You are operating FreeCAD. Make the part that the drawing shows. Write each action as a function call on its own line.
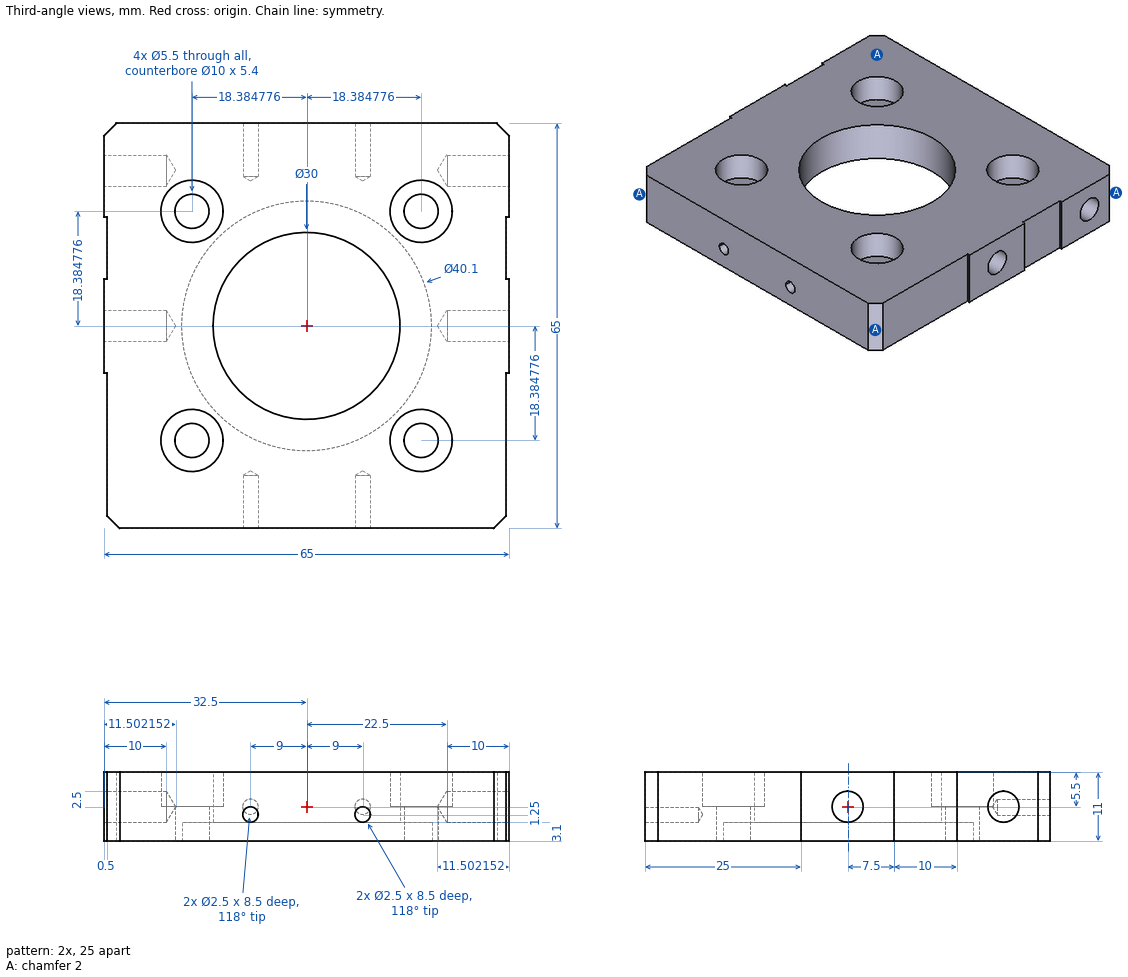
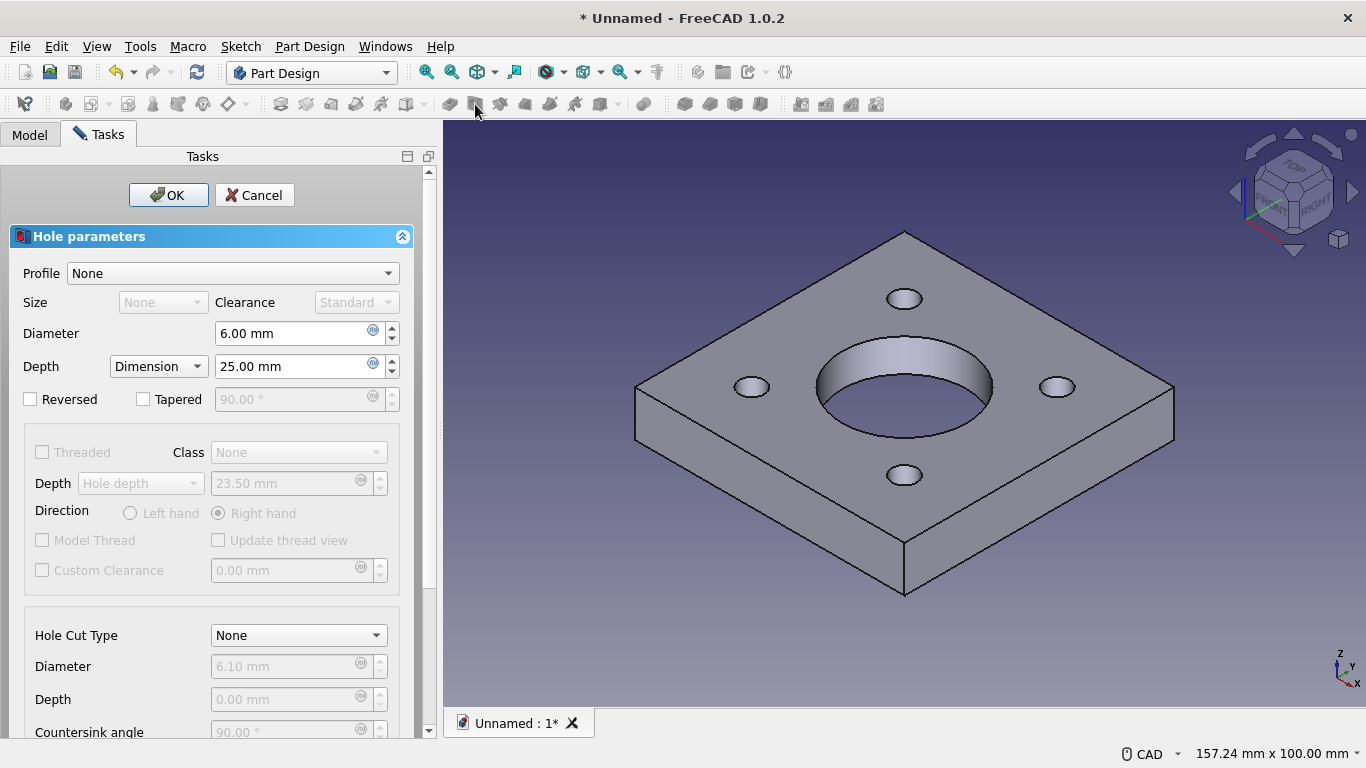
triple_click(300, 334)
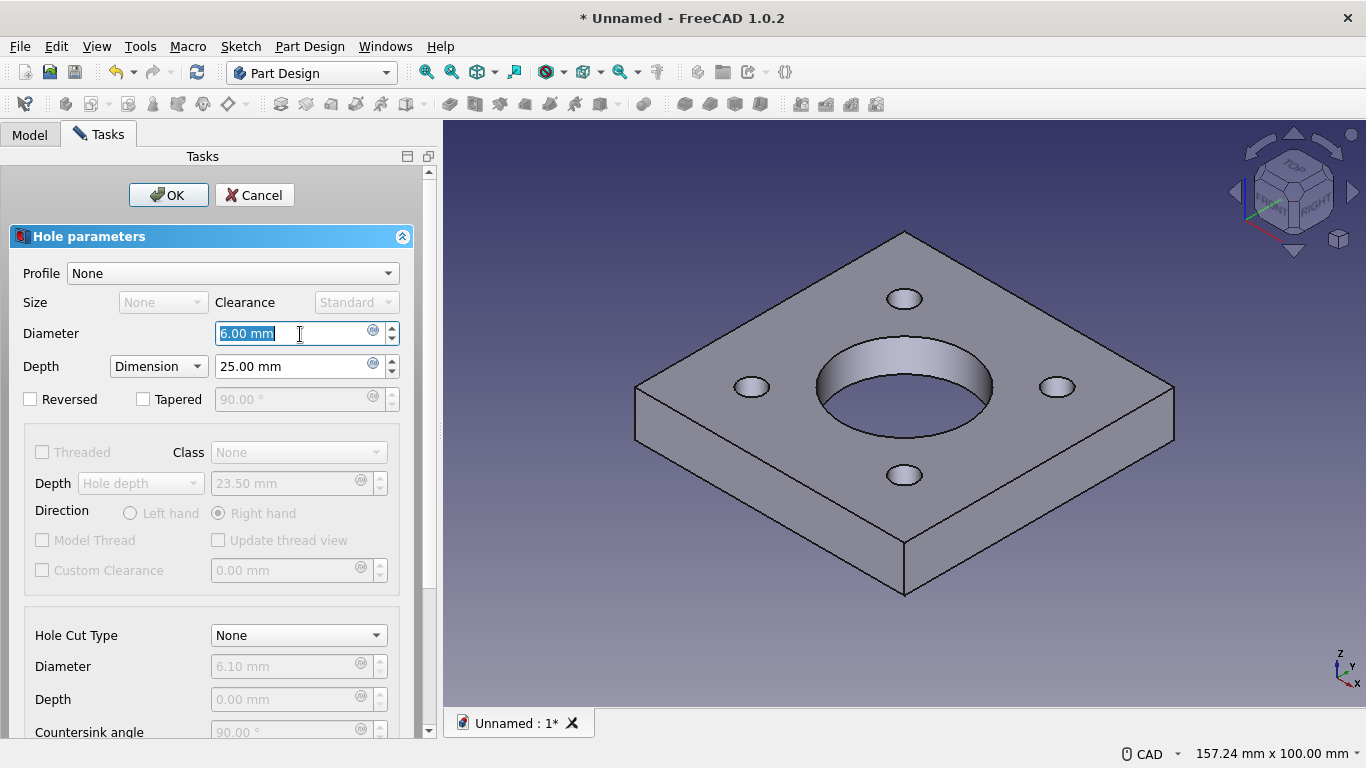
text(5.5)
key(Tab)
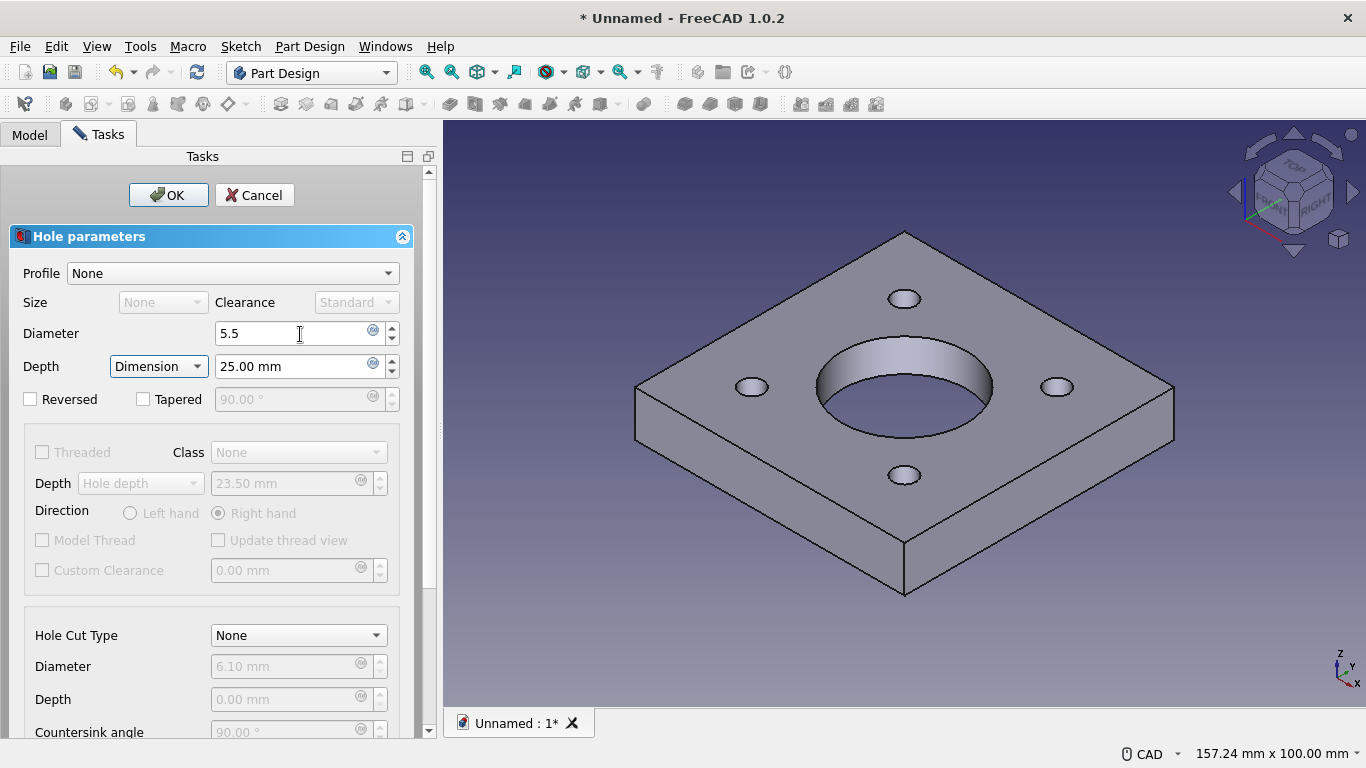
click(160, 366)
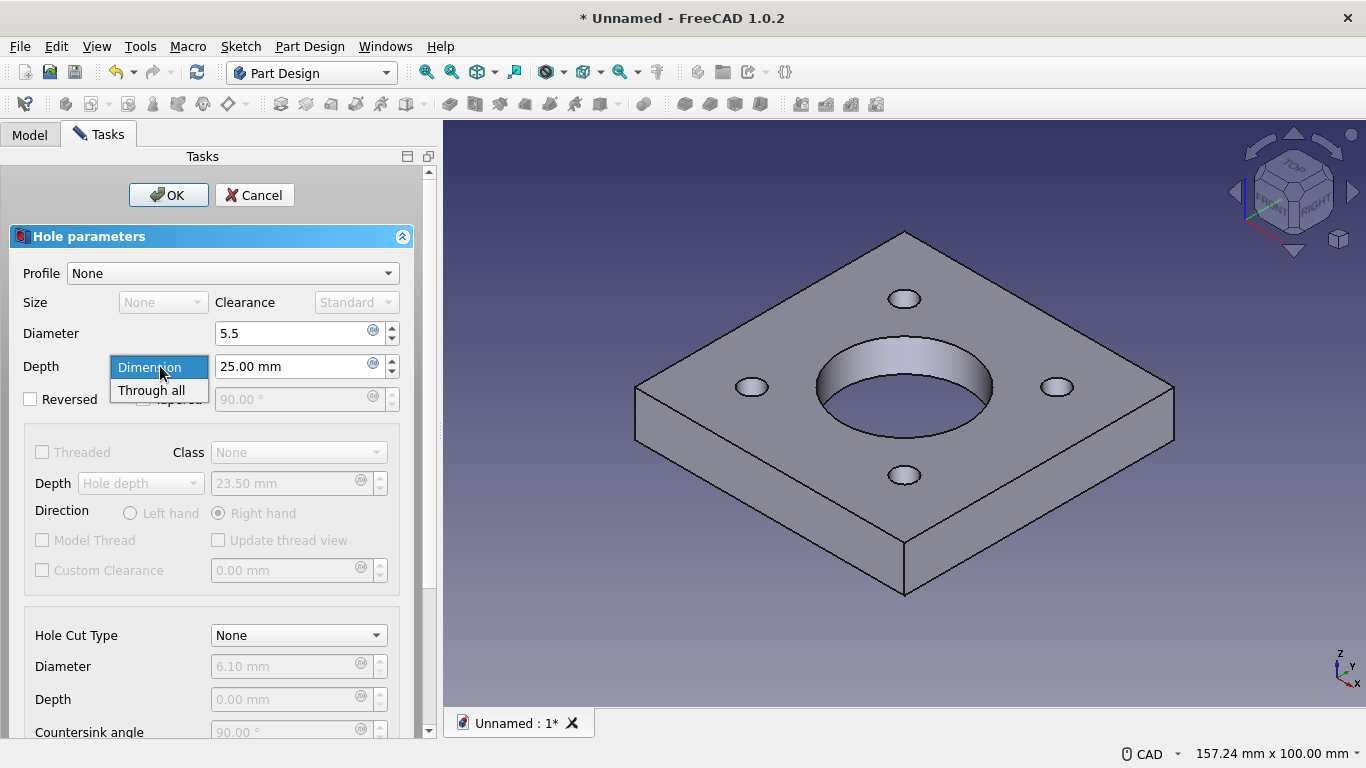
click(158, 390)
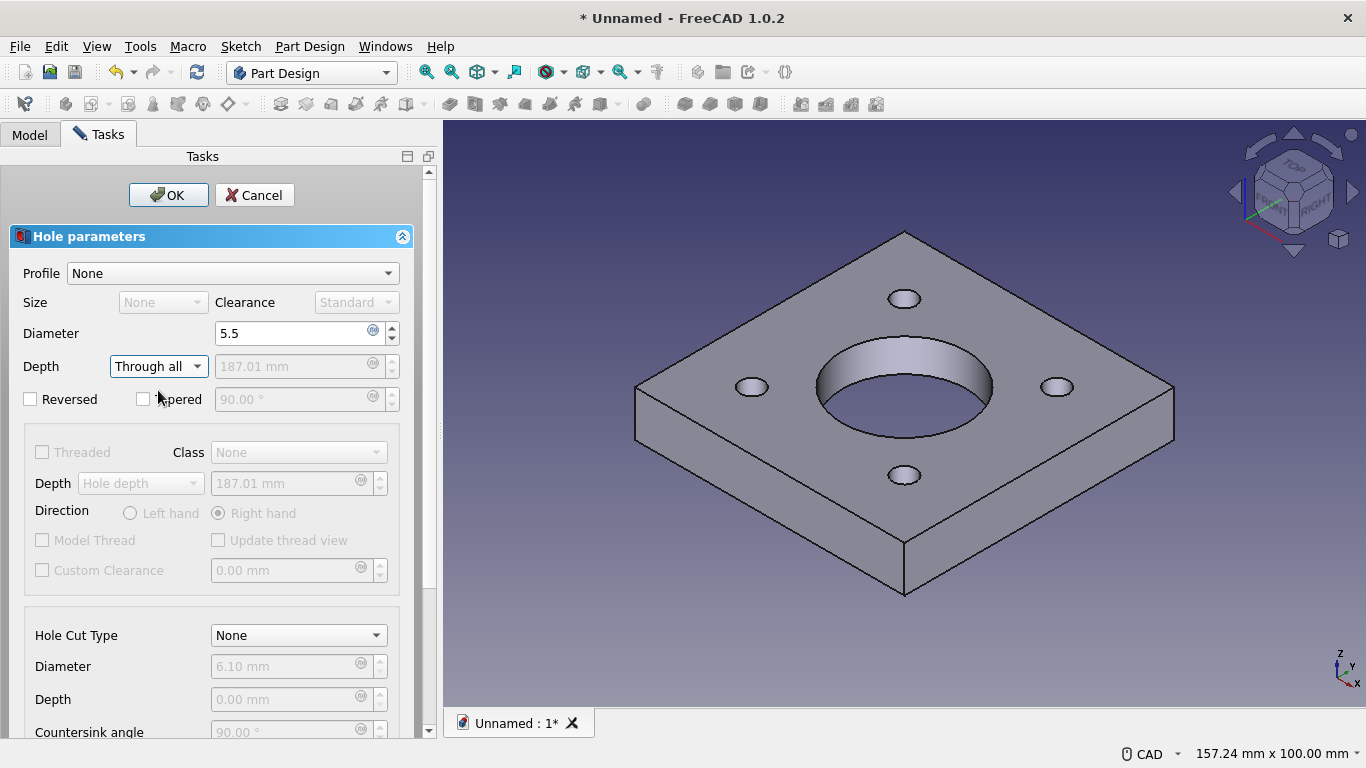
click(300, 636)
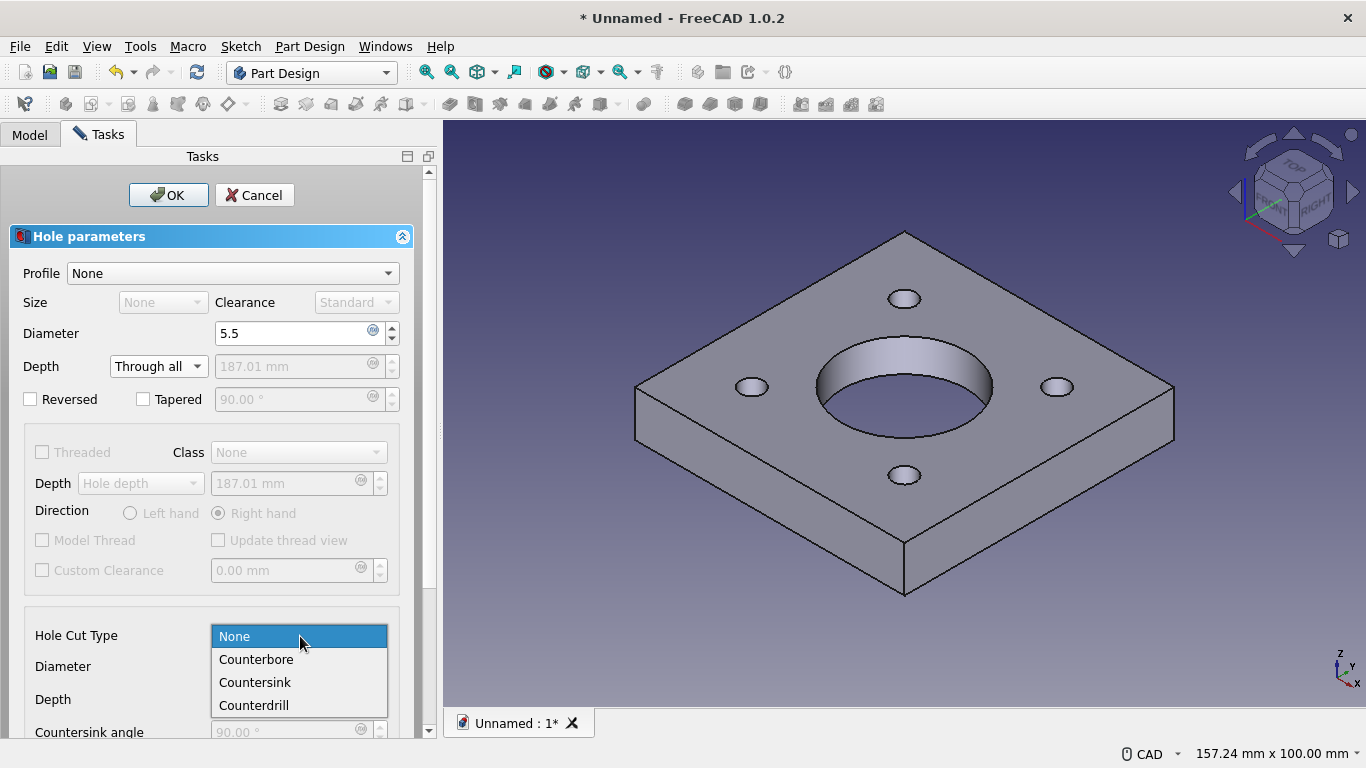
click(298, 660)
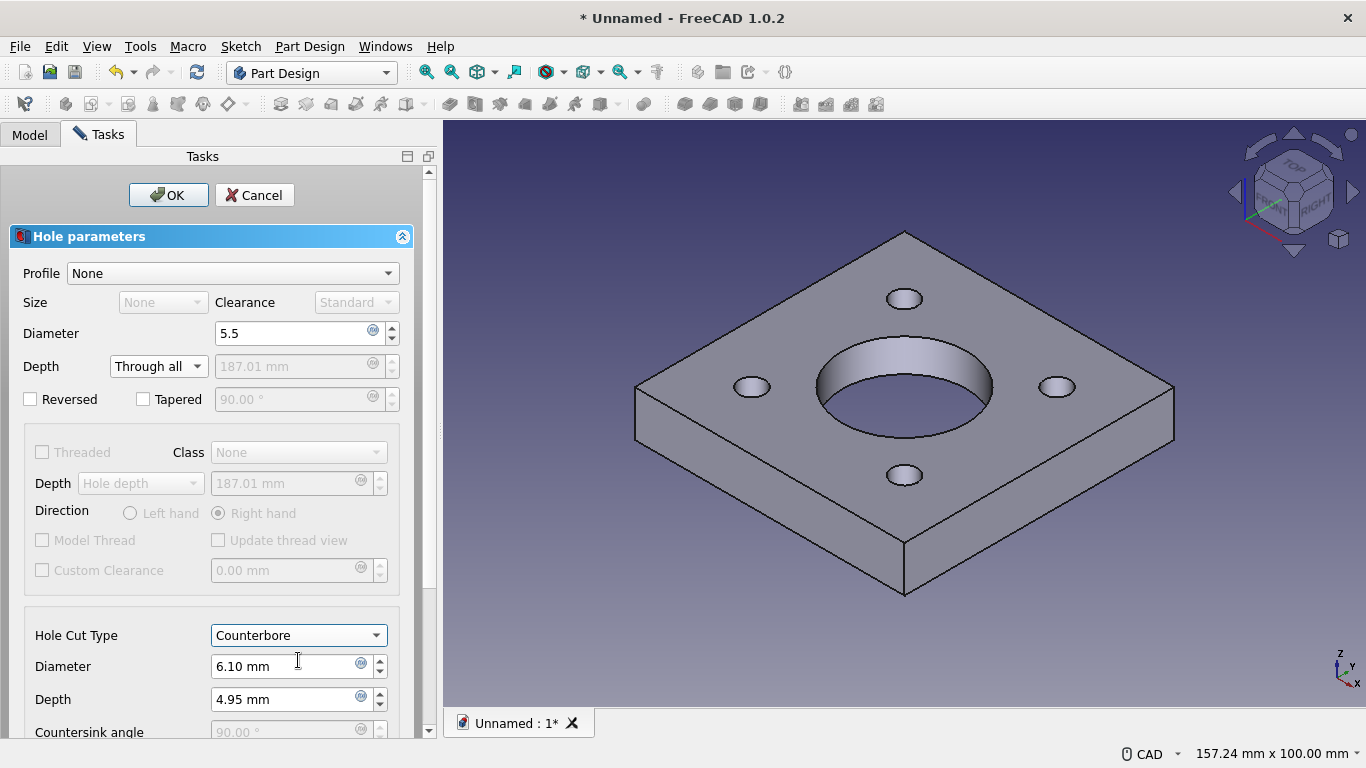
triple_click(292, 666)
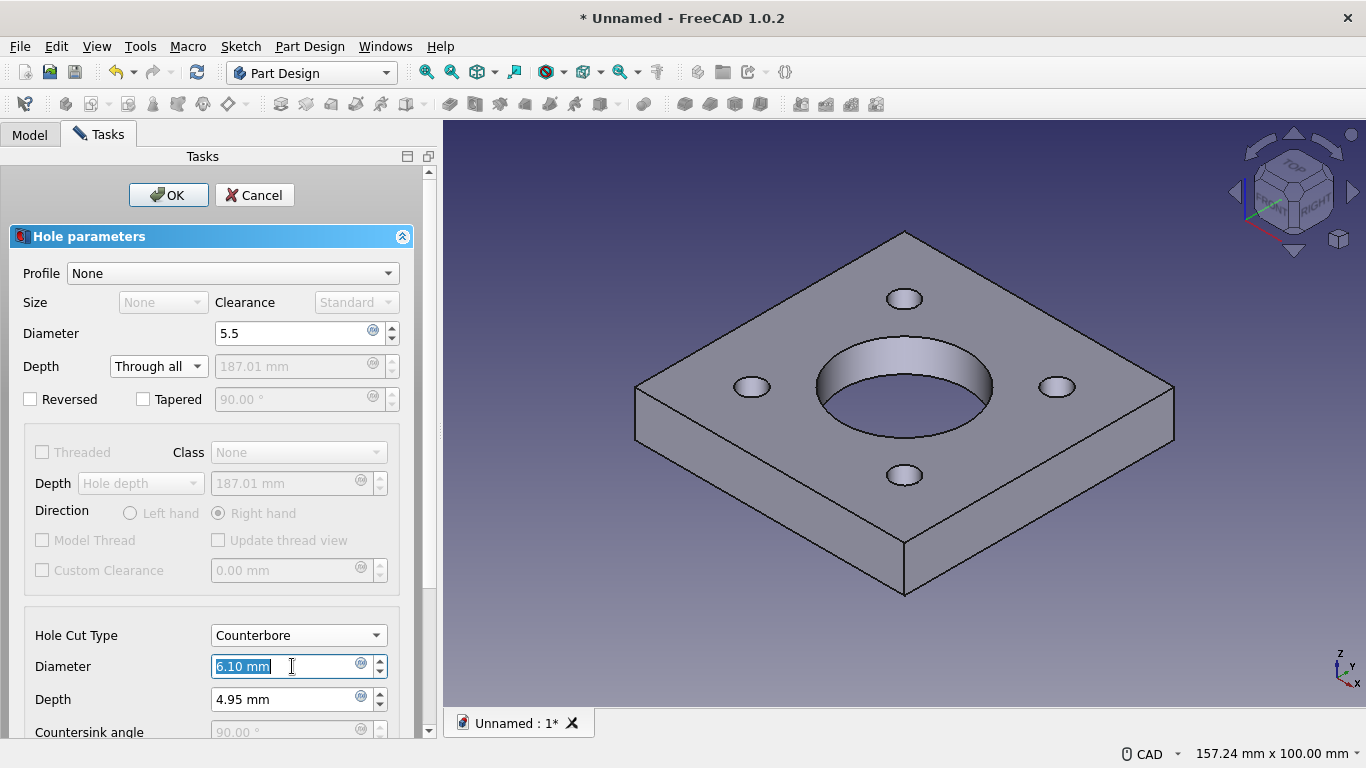
text(10)
key(Tab)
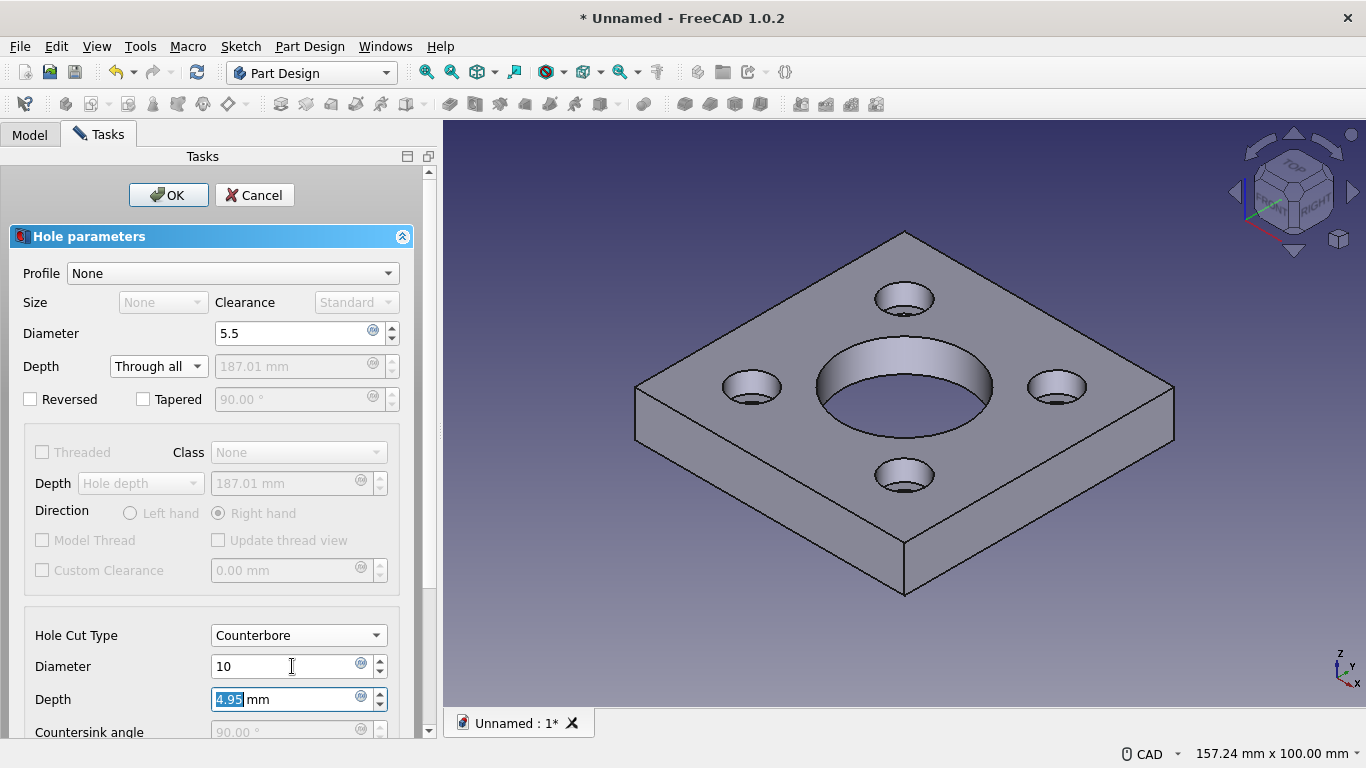
text(5.4)
key(Tab)